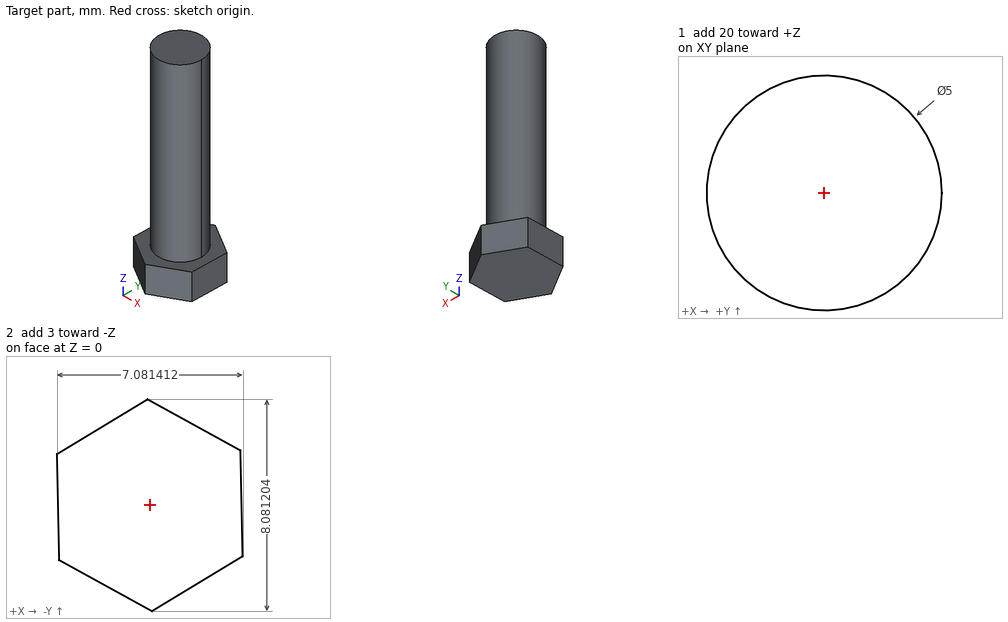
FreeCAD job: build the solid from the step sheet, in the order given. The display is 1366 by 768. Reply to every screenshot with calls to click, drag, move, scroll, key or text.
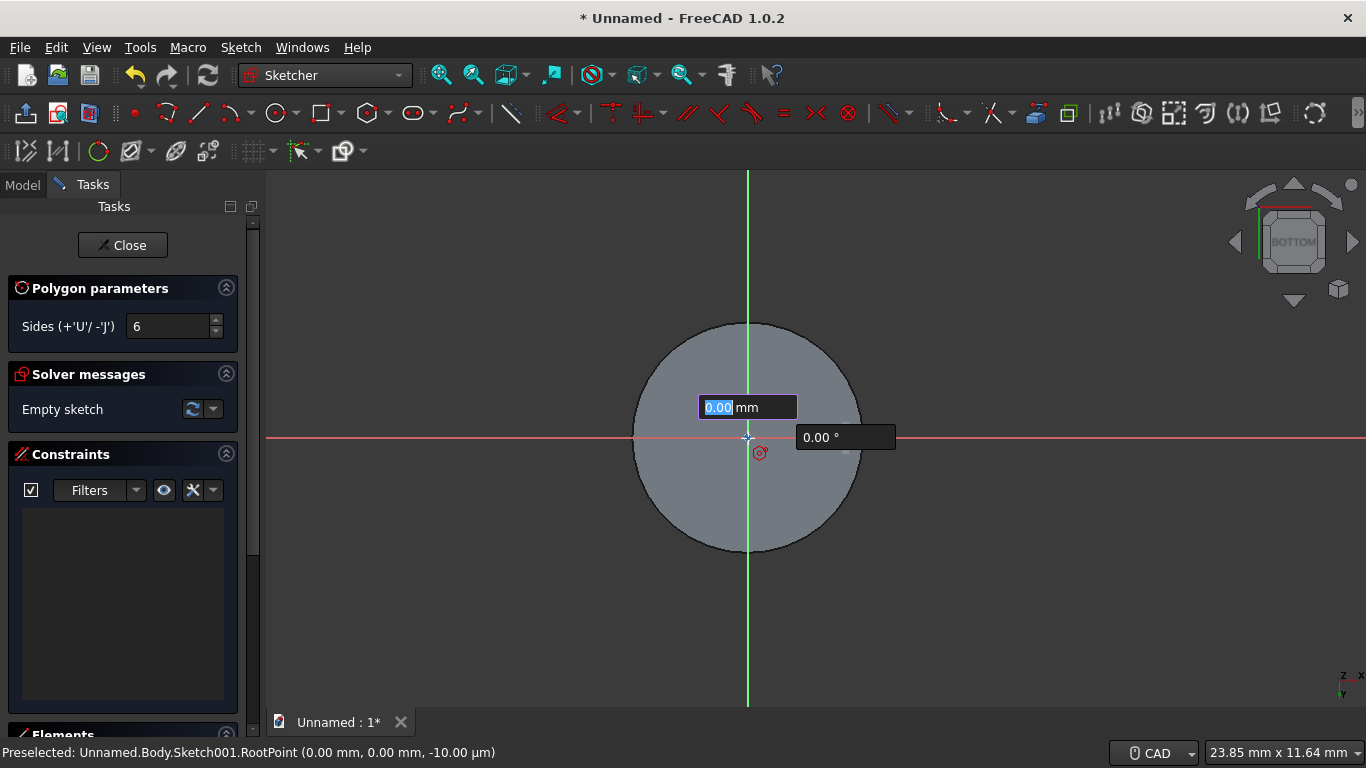
click(588, 534)
key(Escape)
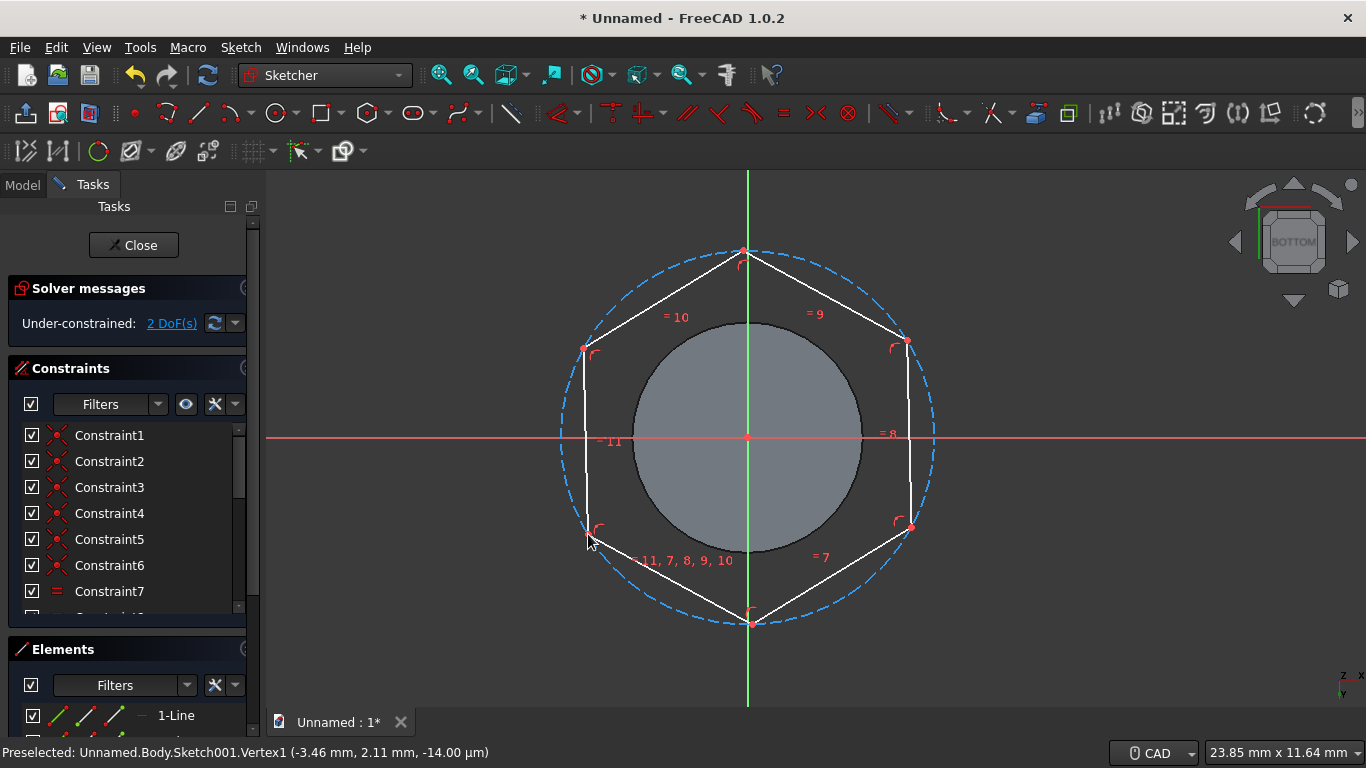
click(558, 114)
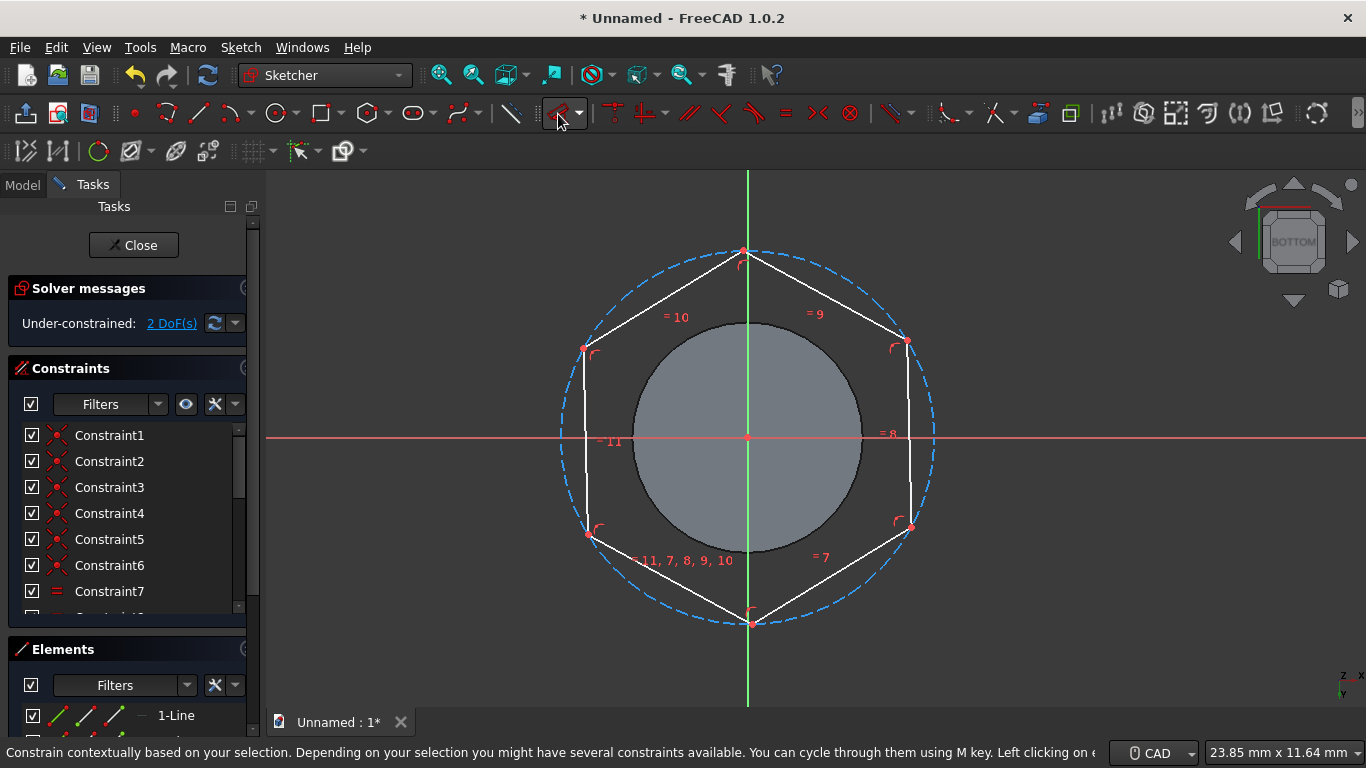
click(752, 625)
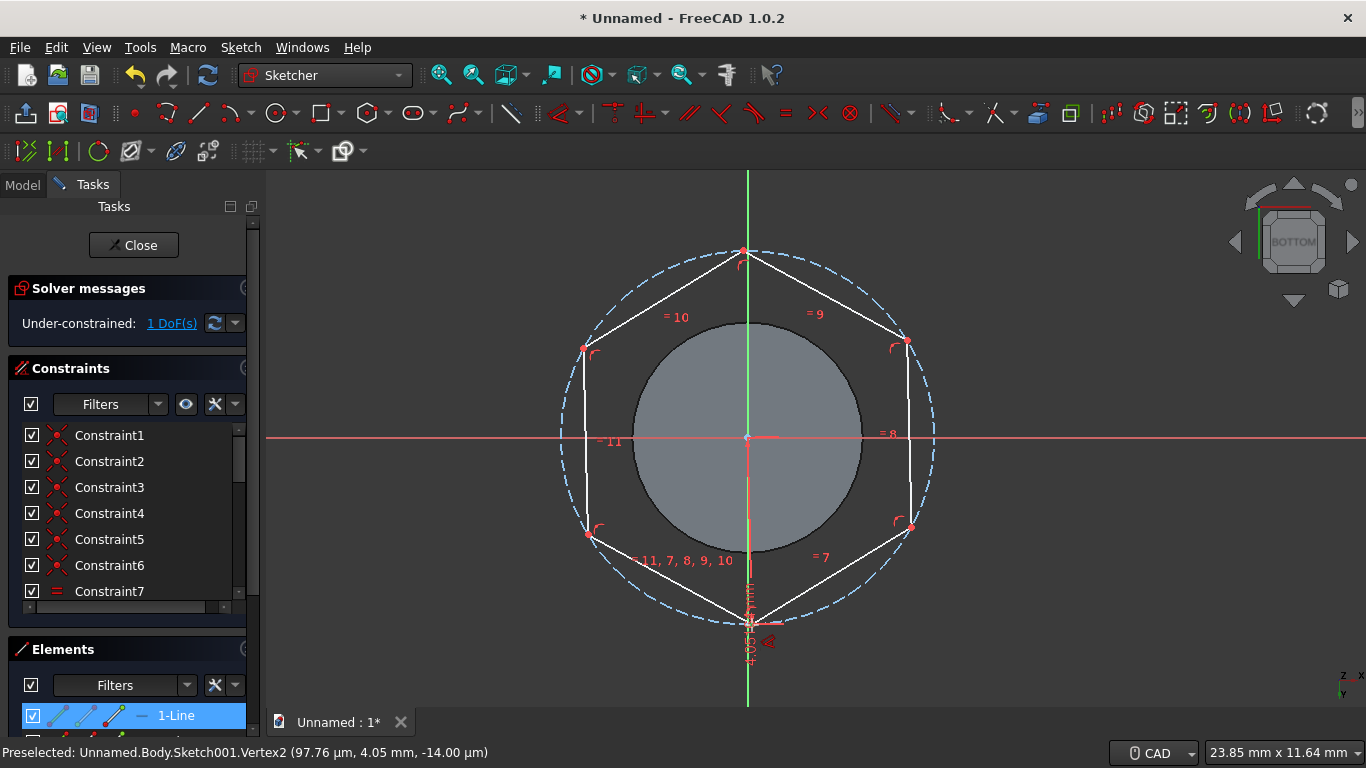
click(743, 251)
click(786, 352)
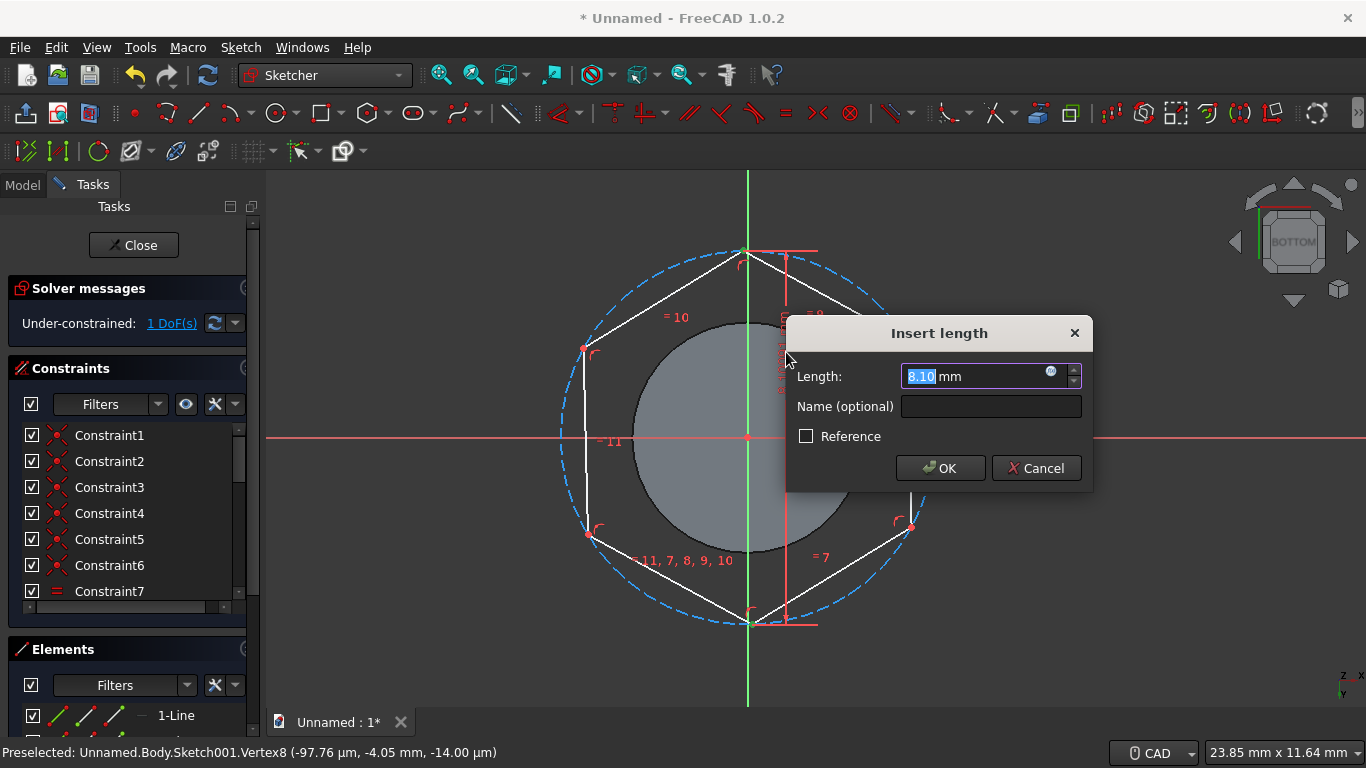
text(8.081204)
key(Return)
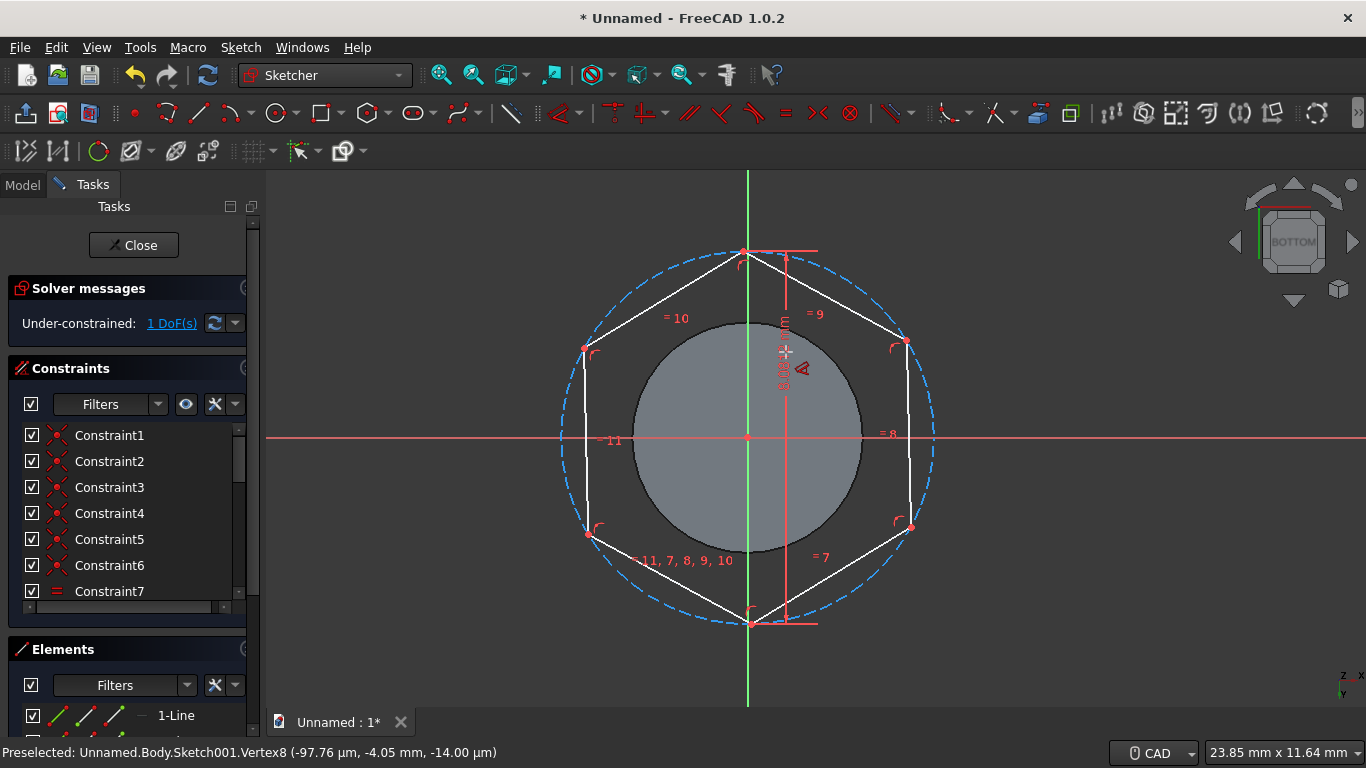
click(584, 348)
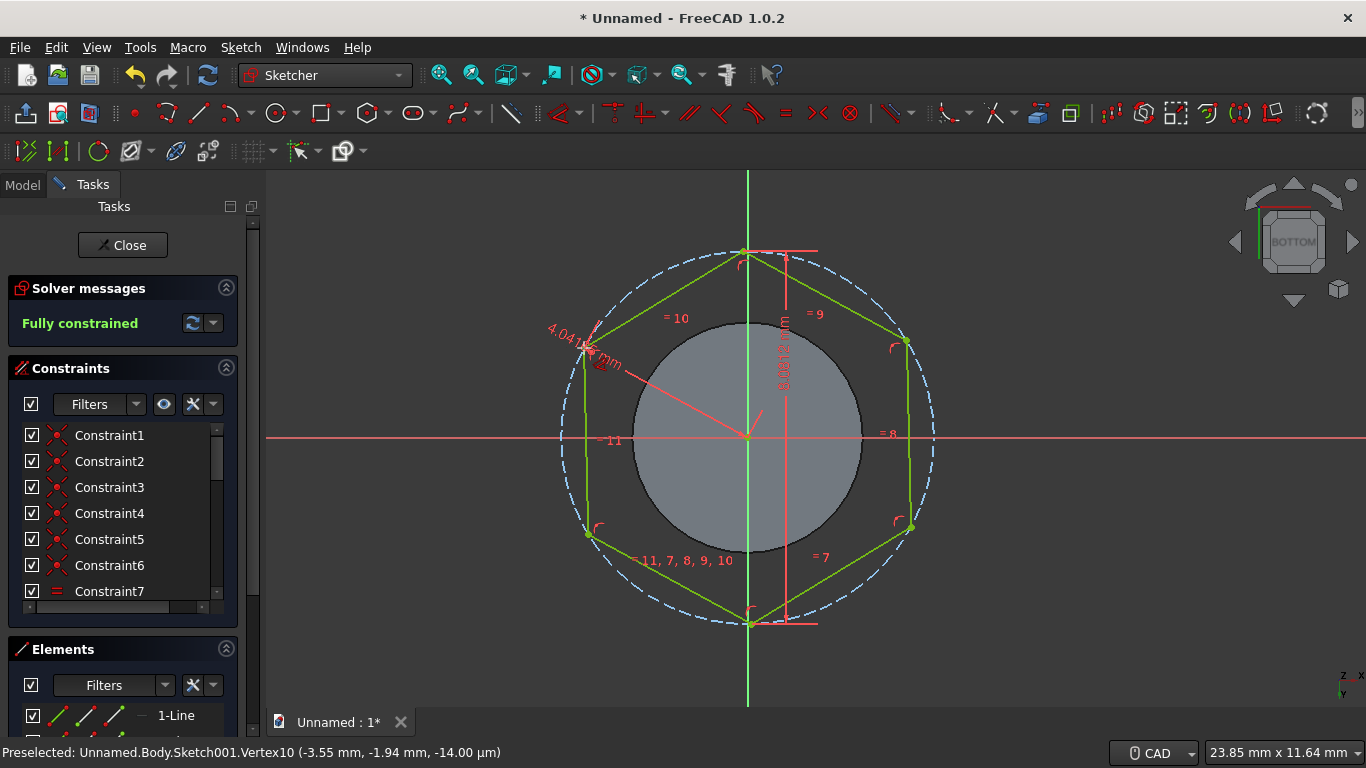
click(911, 527)
click(672, 561)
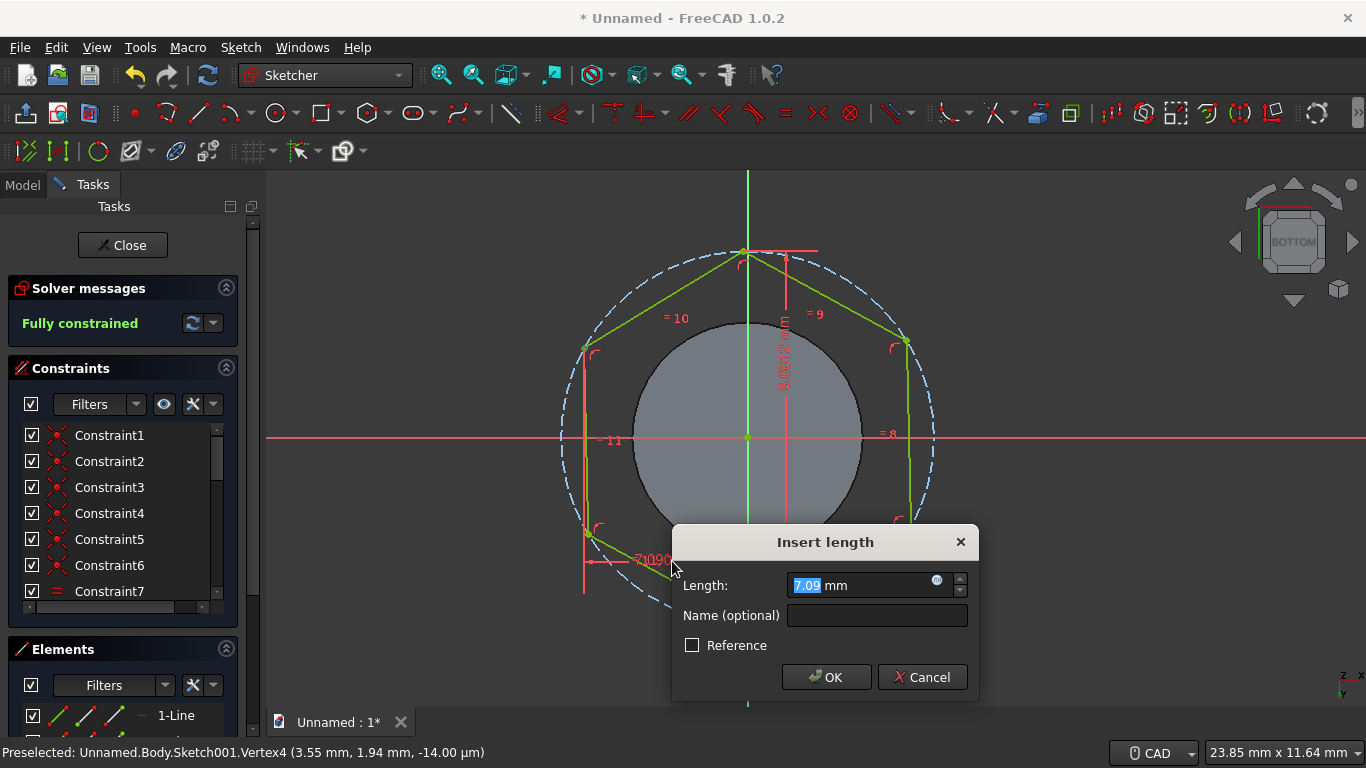
text(7.081412)
key(Return)
key(Escape)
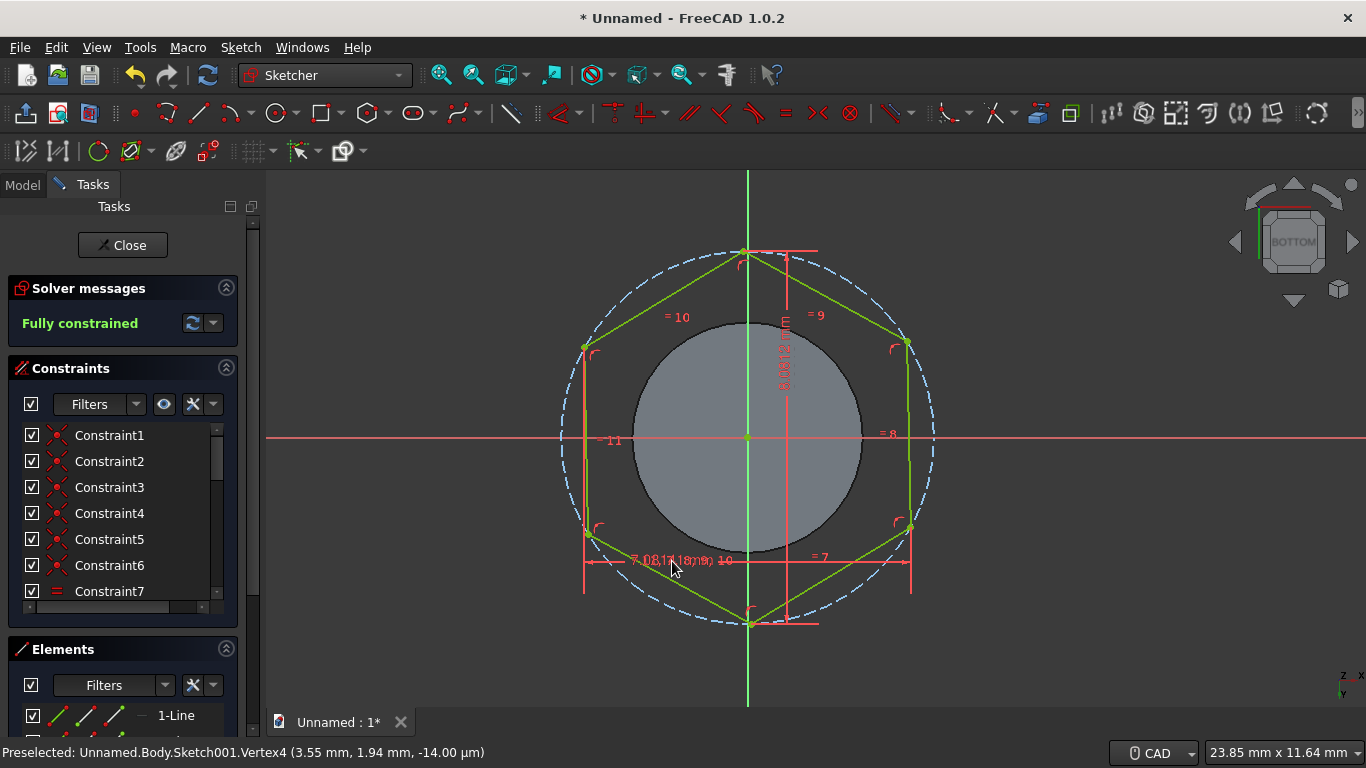
click(123, 245)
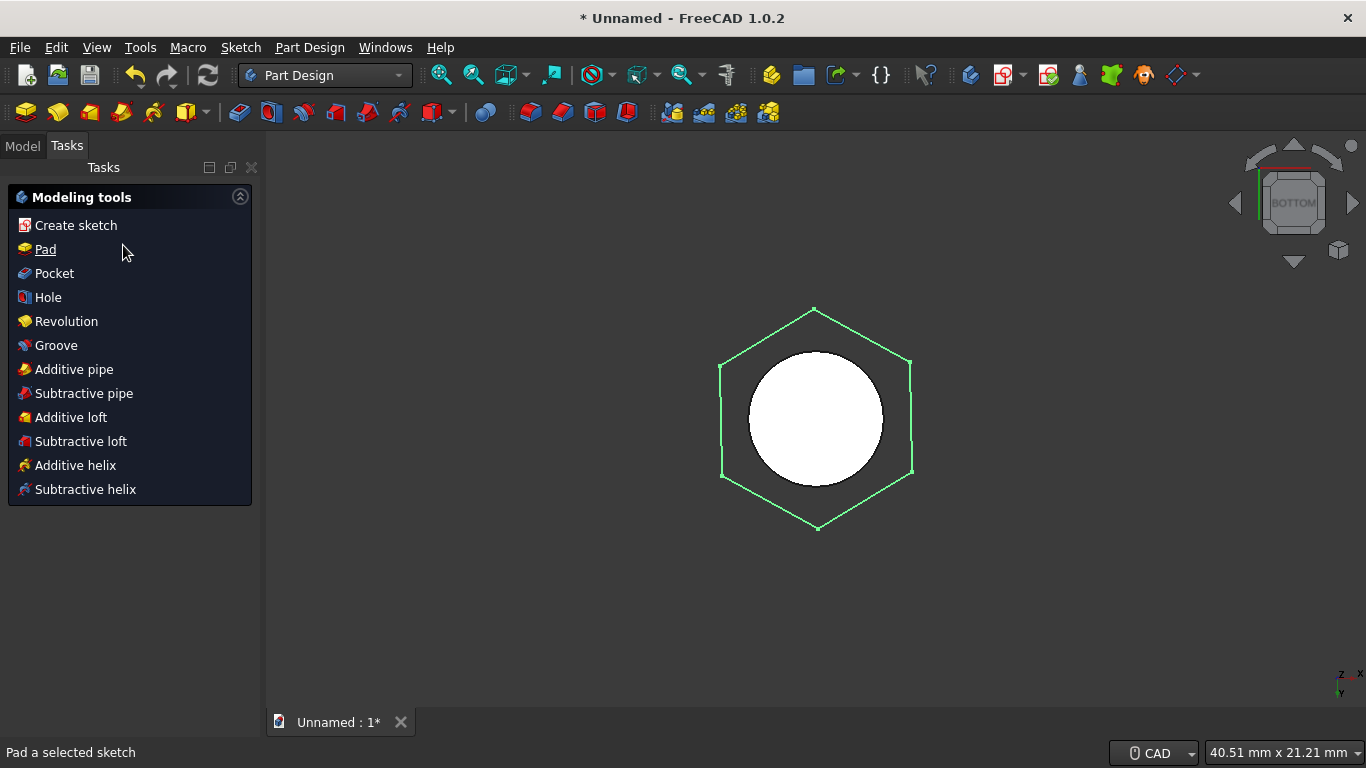
click(26, 112)